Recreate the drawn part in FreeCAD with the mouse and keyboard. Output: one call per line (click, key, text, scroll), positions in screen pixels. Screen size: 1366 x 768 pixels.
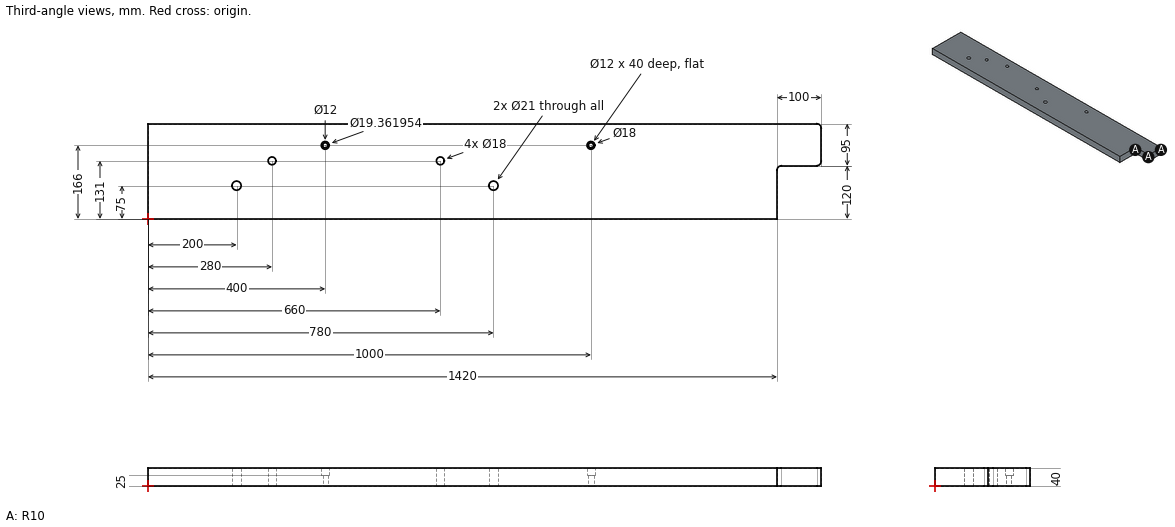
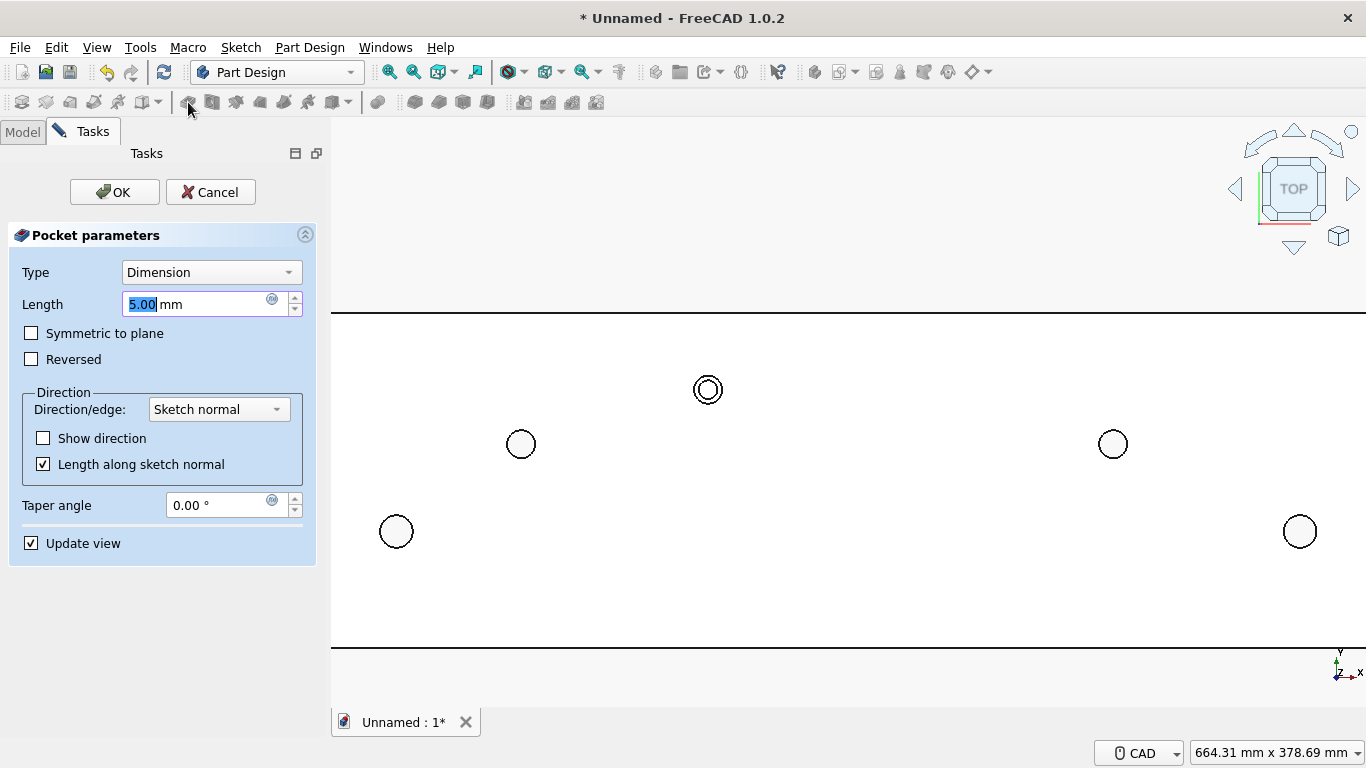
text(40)
key(Tab)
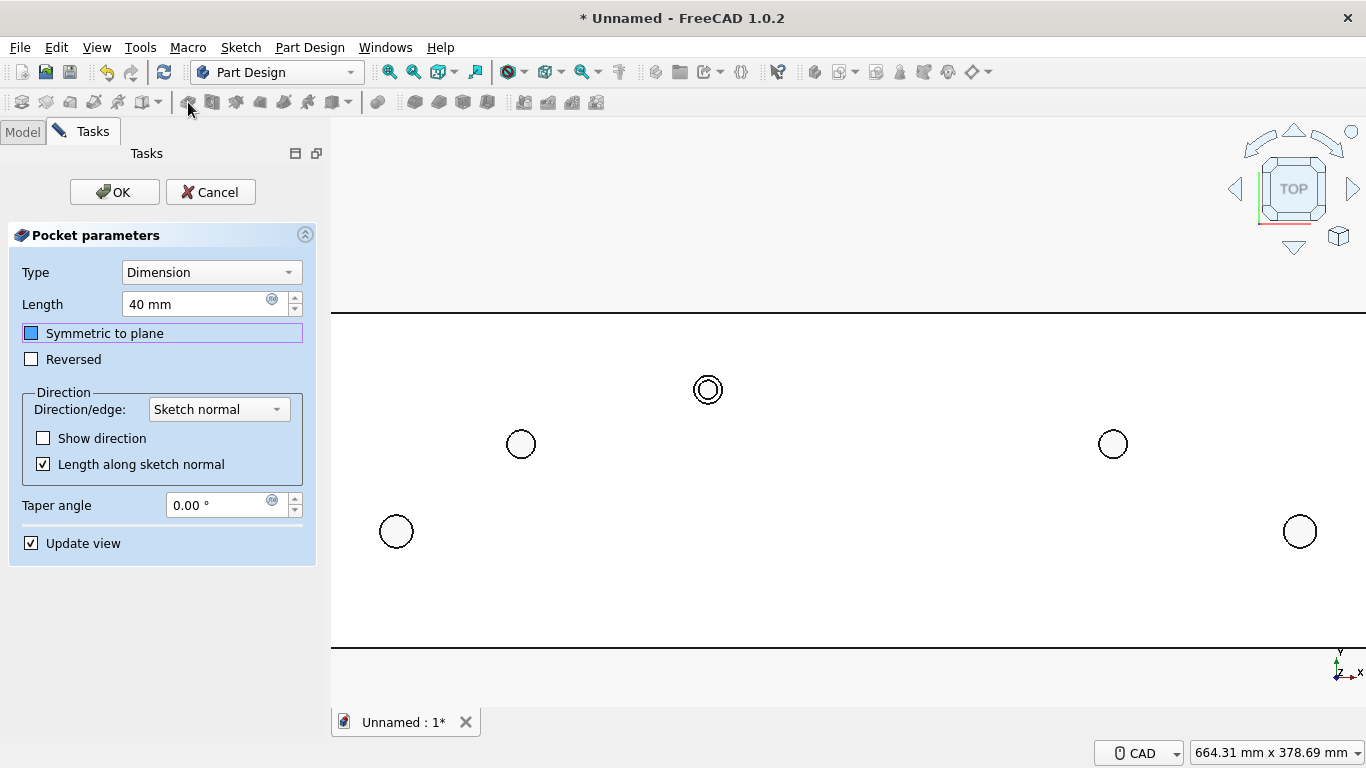
click(115, 192)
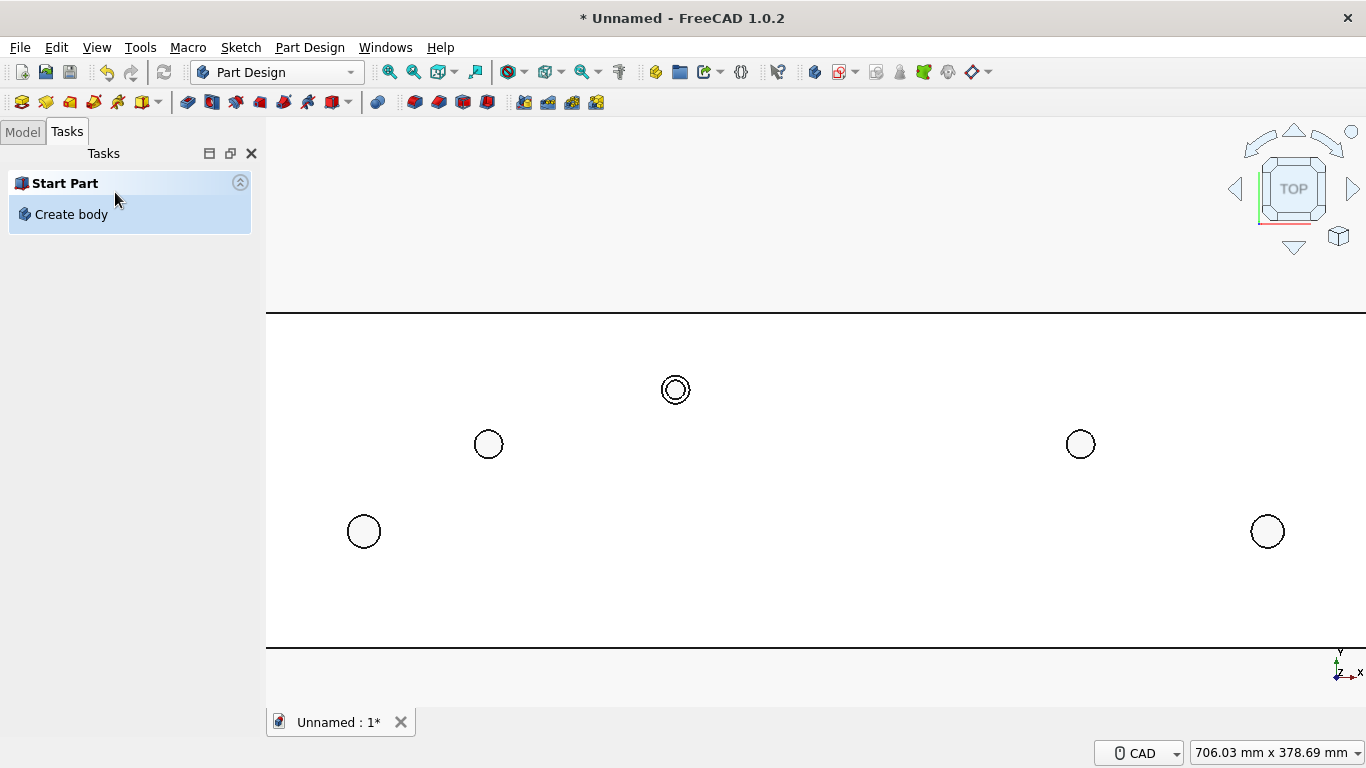
key(0)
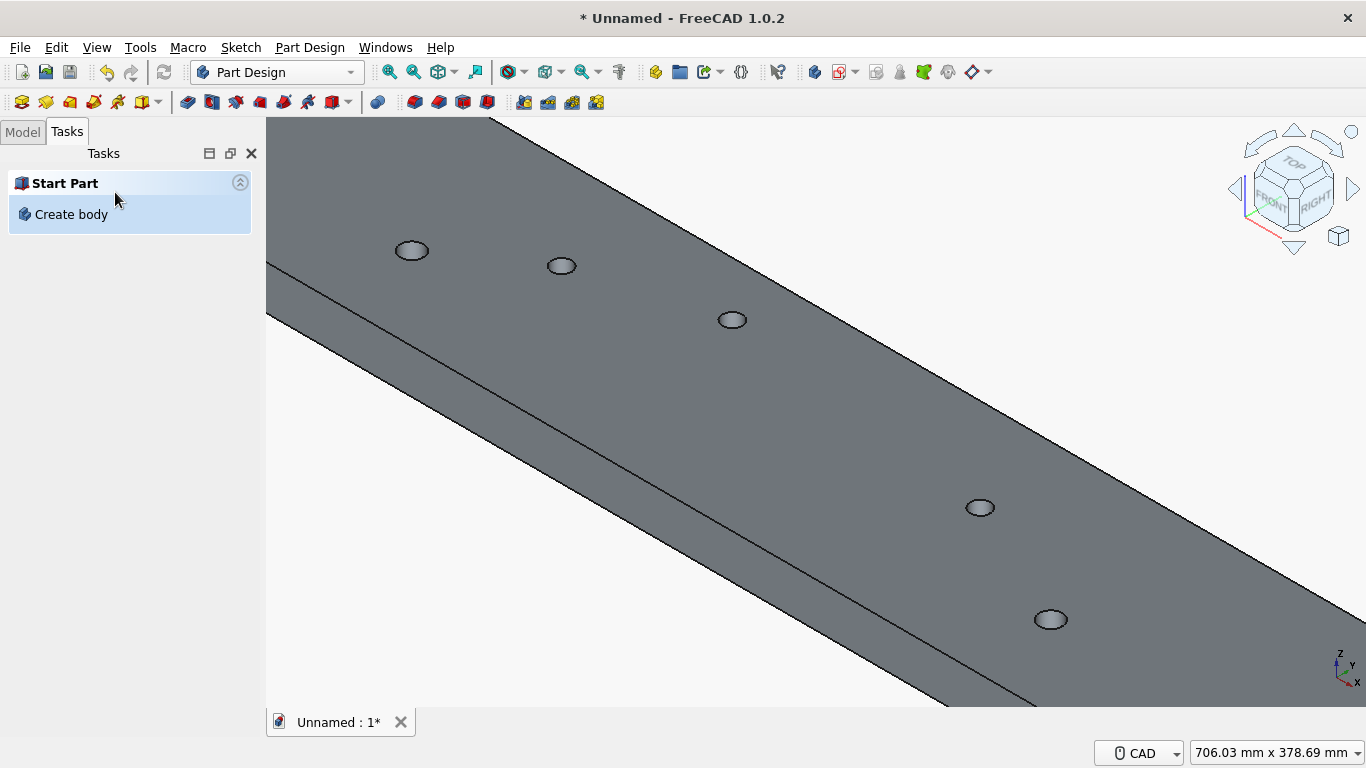
key(v)
key(f)